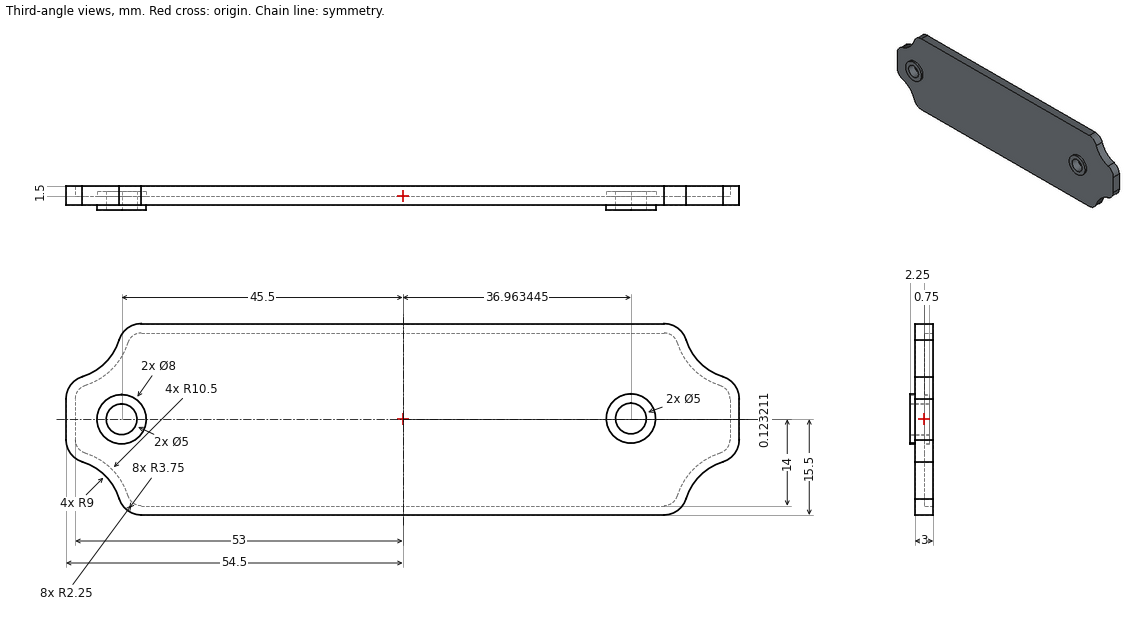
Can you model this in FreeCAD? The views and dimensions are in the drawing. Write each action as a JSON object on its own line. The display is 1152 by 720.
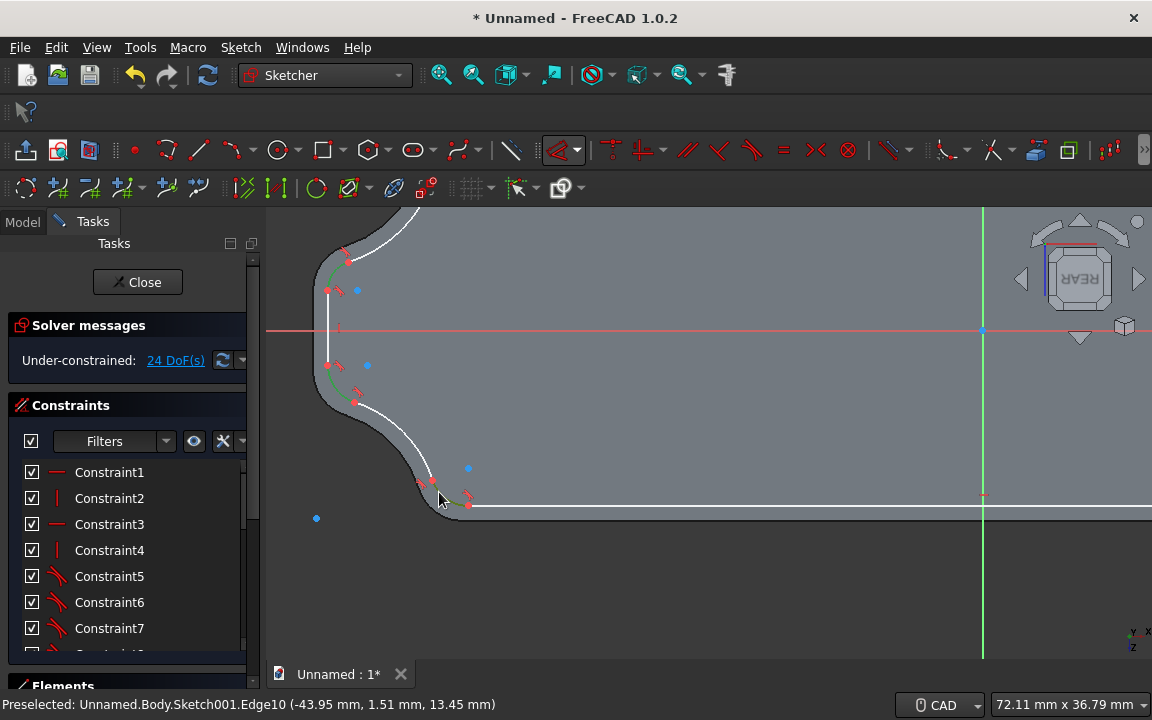
{"action": "scroll", "coordinate": [441, 493], "scroll_direction": "down", "scroll_amount": 5}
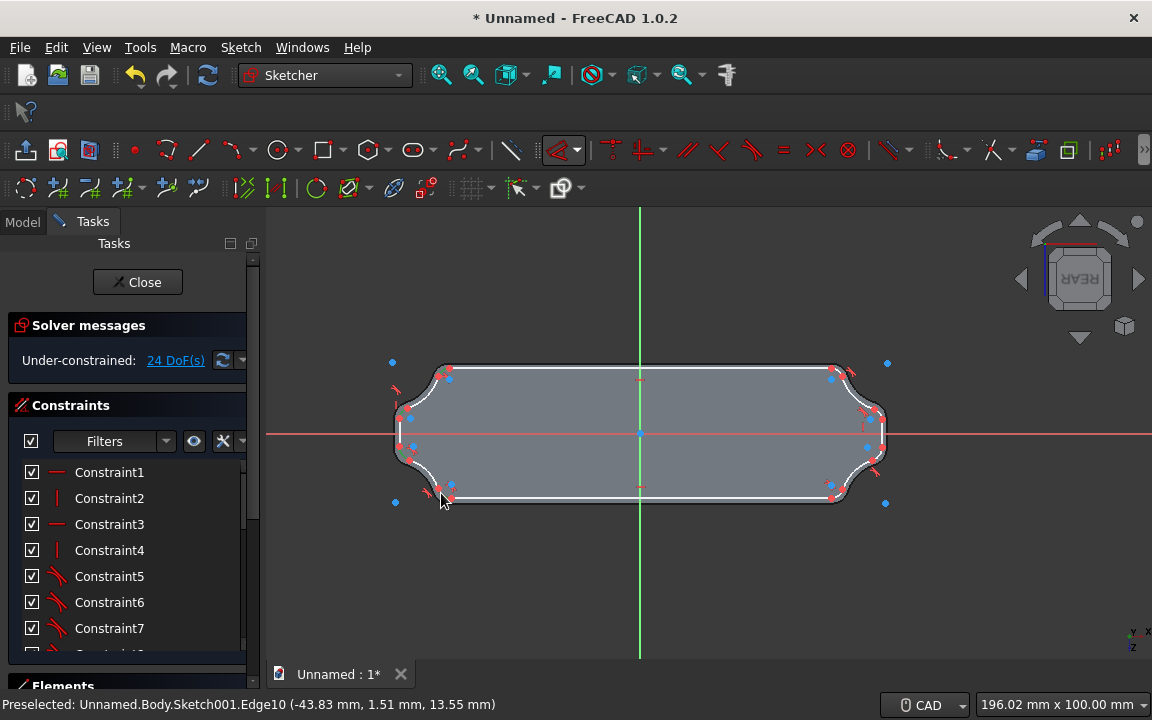
{"action": "scroll", "coordinate": [836, 497], "scroll_direction": "up", "scroll_amount": 6}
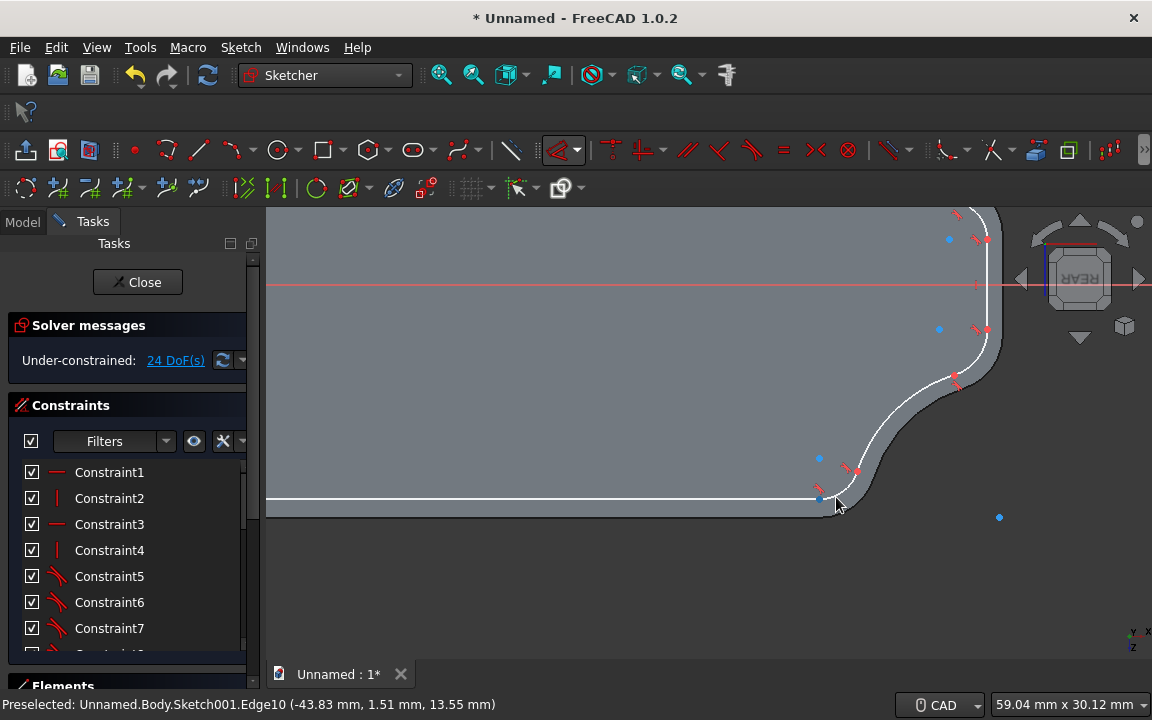
{"action": "left_click", "coordinate": [834, 497]}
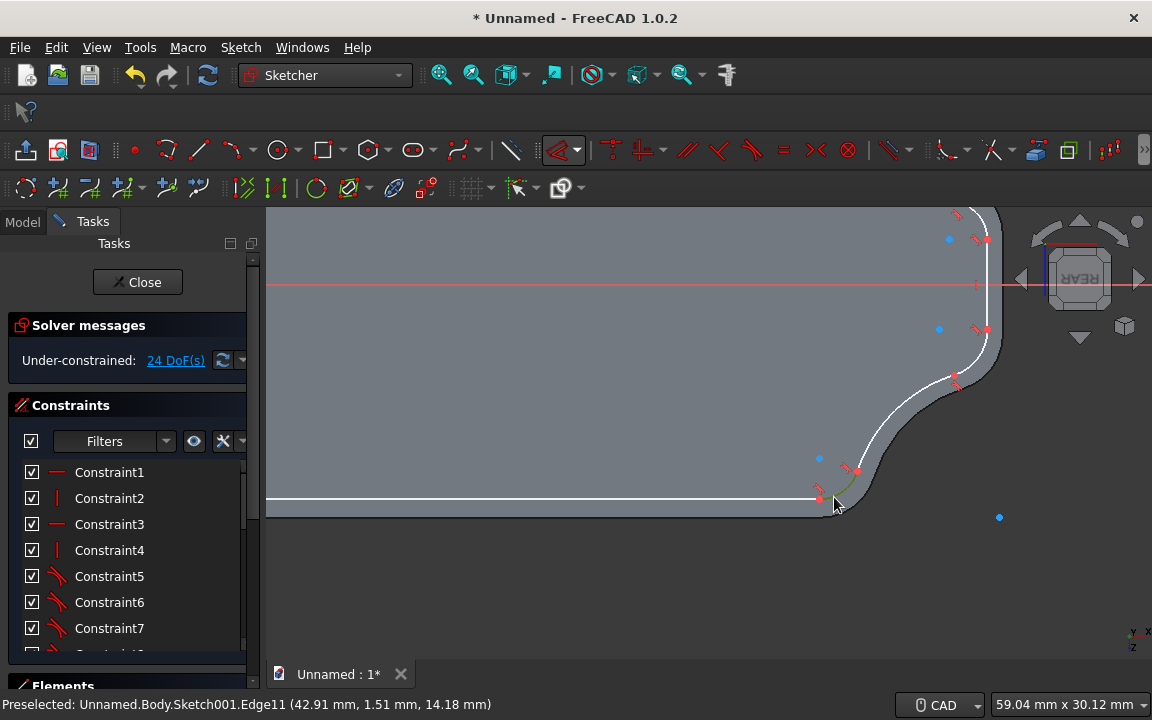
{"action": "left_click", "coordinate": [970, 366]}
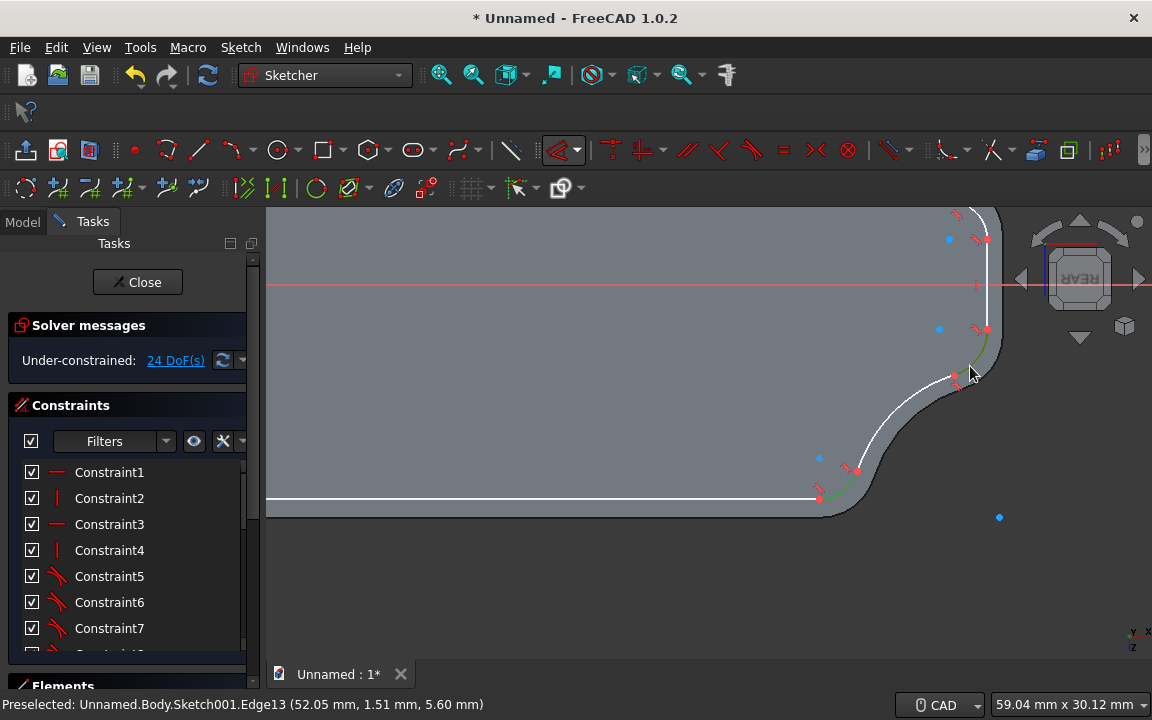
{"action": "scroll", "coordinate": [837, 497], "scroll_direction": "down", "scroll_amount": 6}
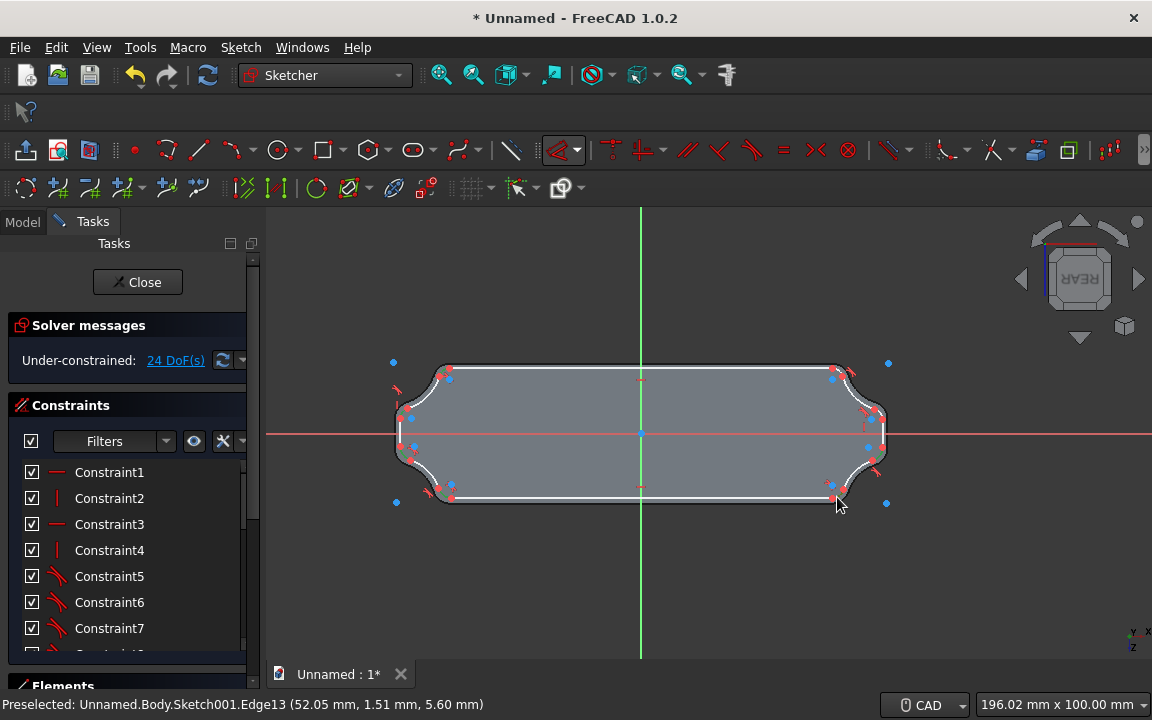
{"action": "scroll", "coordinate": [882, 416], "scroll_direction": "up", "scroll_amount": 6}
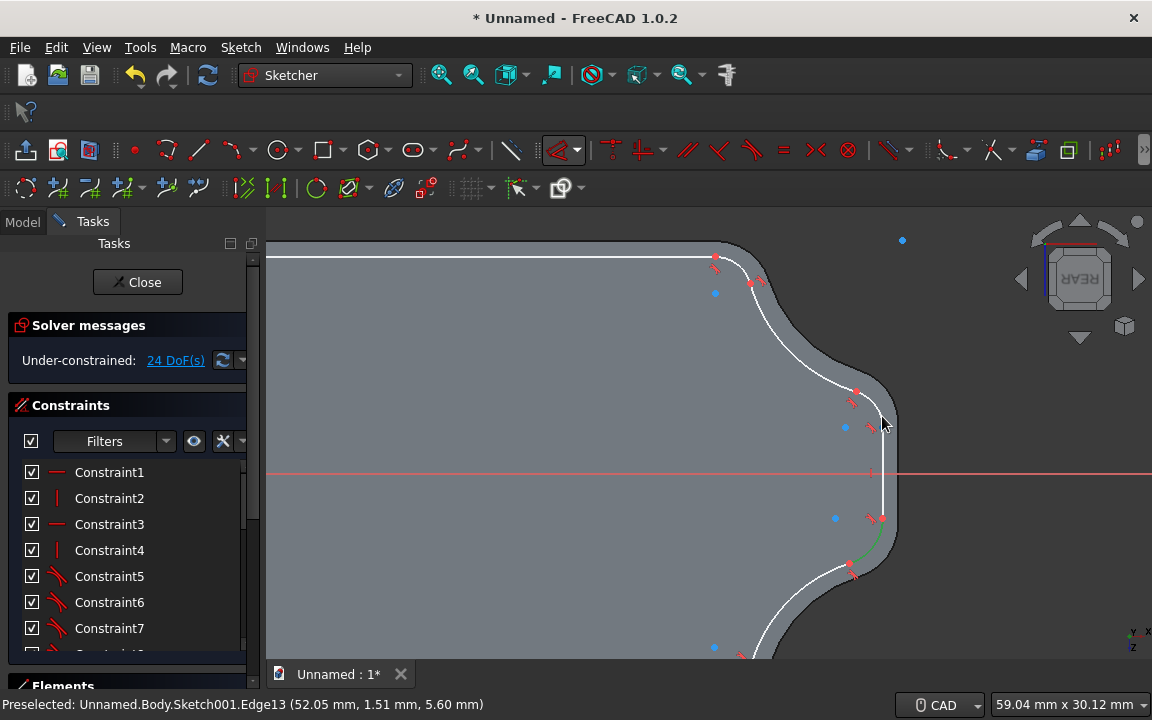
{"action": "left_click", "coordinate": [880, 414]}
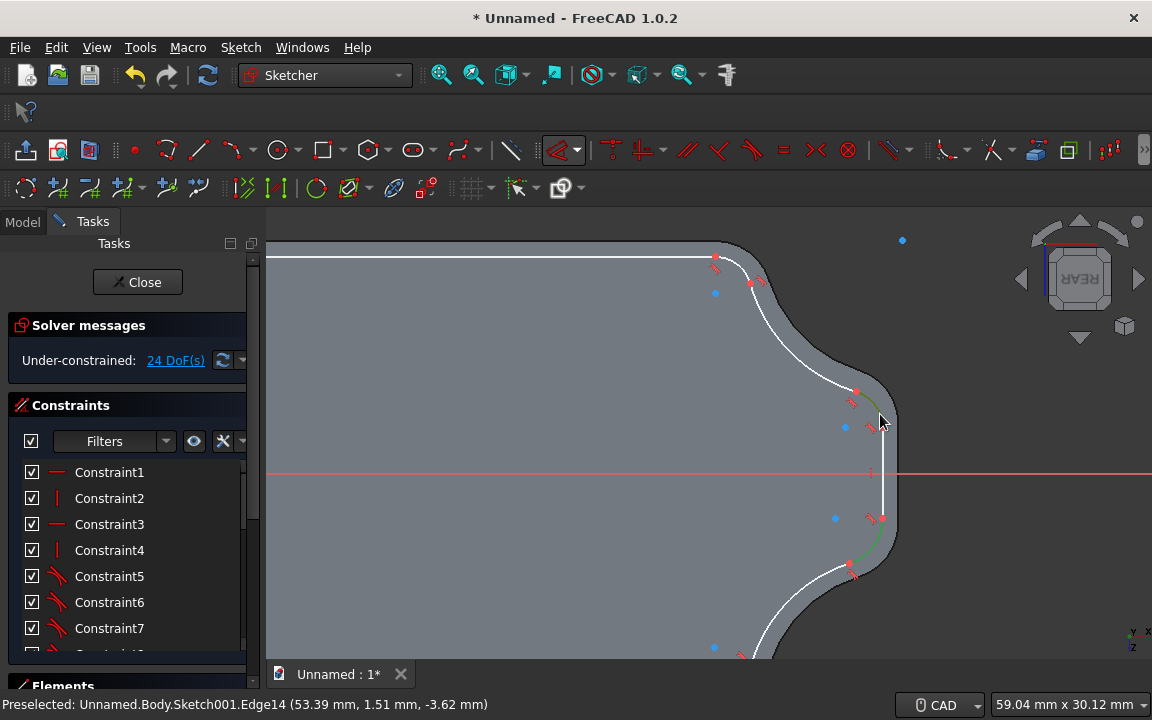
{"action": "left_click", "coordinate": [744, 271]}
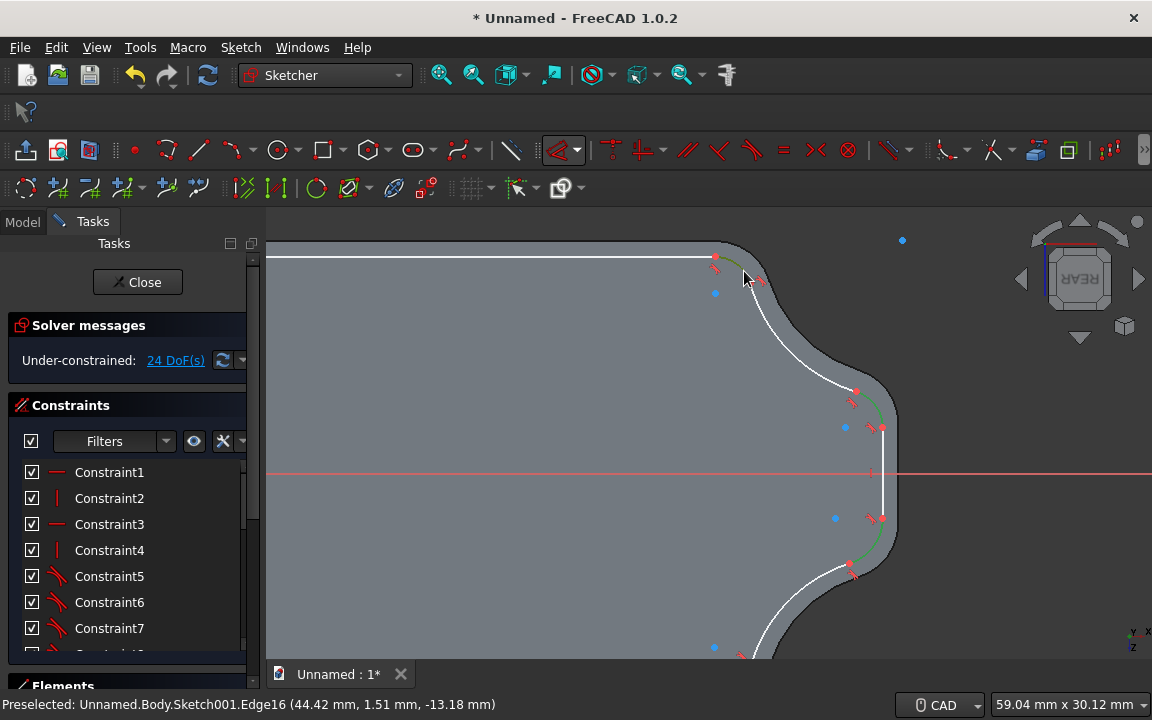
{"action": "left_click", "coordinate": [784, 150]}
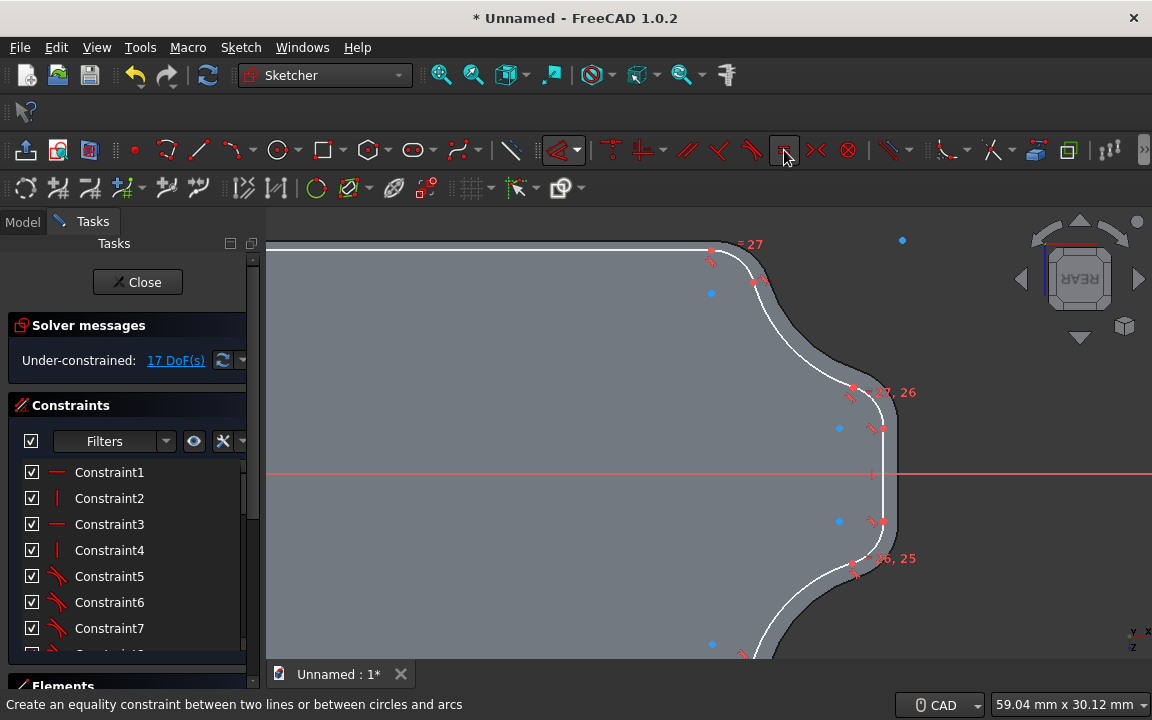
{"action": "scroll", "coordinate": [882, 416], "scroll_direction": "down", "scroll_amount": 6}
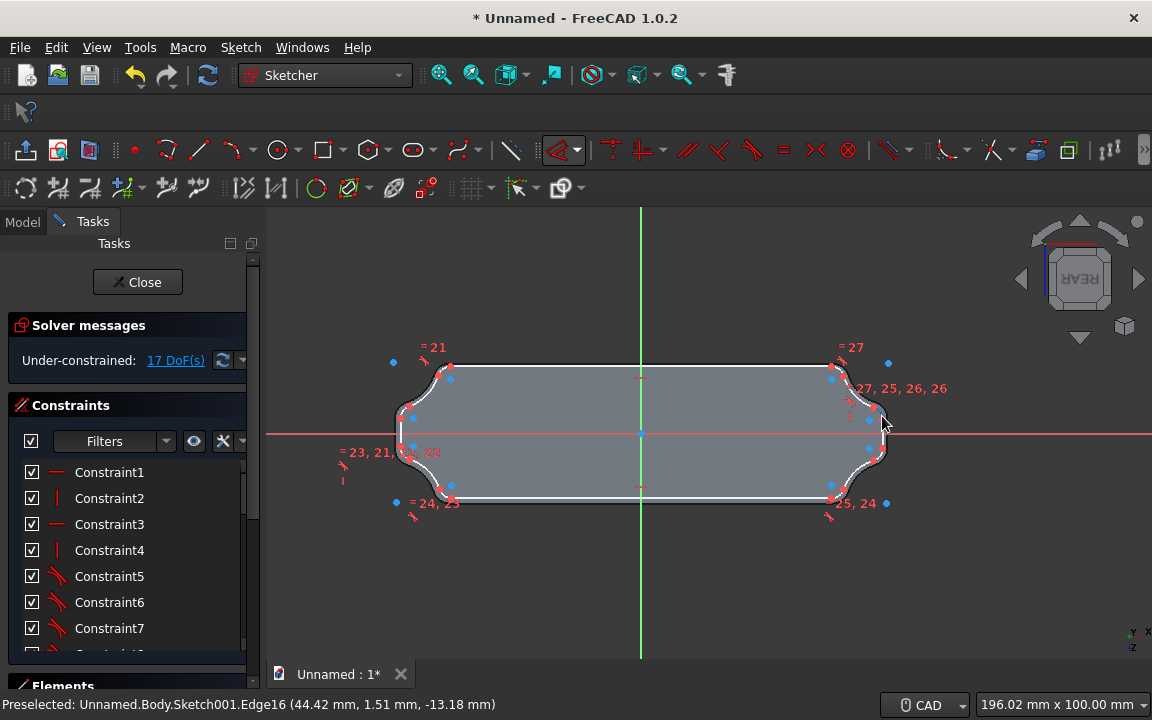
{"action": "left_click", "coordinate": [421, 400]}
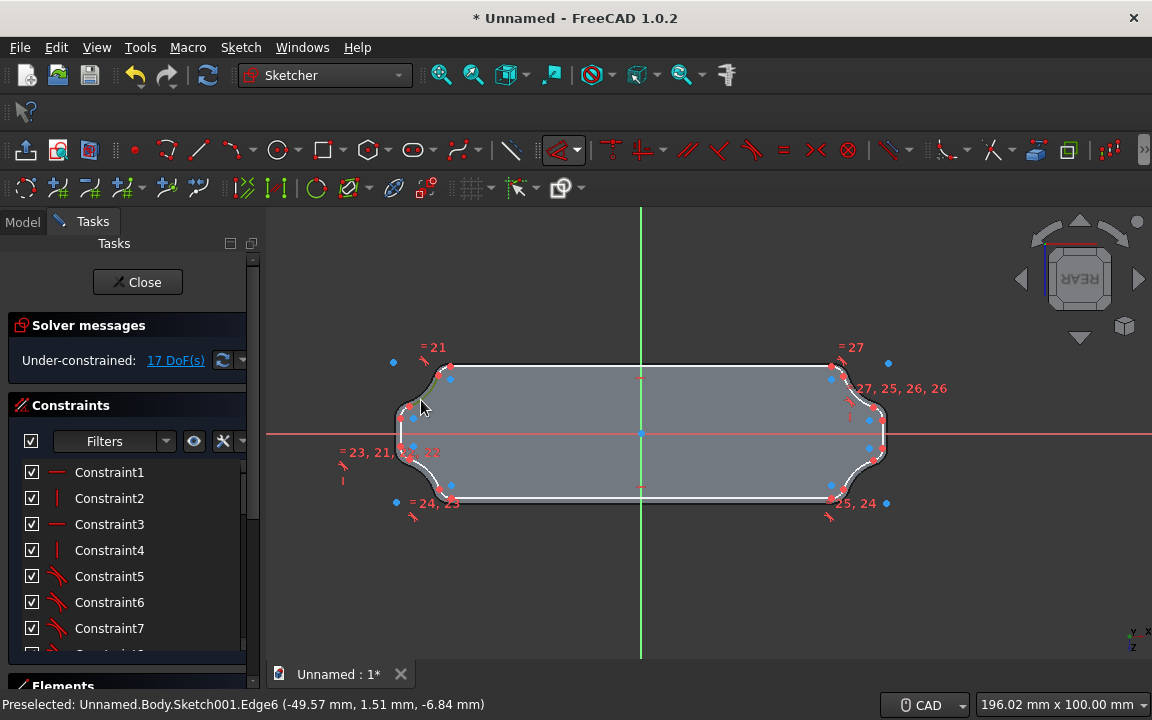
{"action": "scroll", "coordinate": [434, 477], "scroll_direction": "up", "scroll_amount": 4}